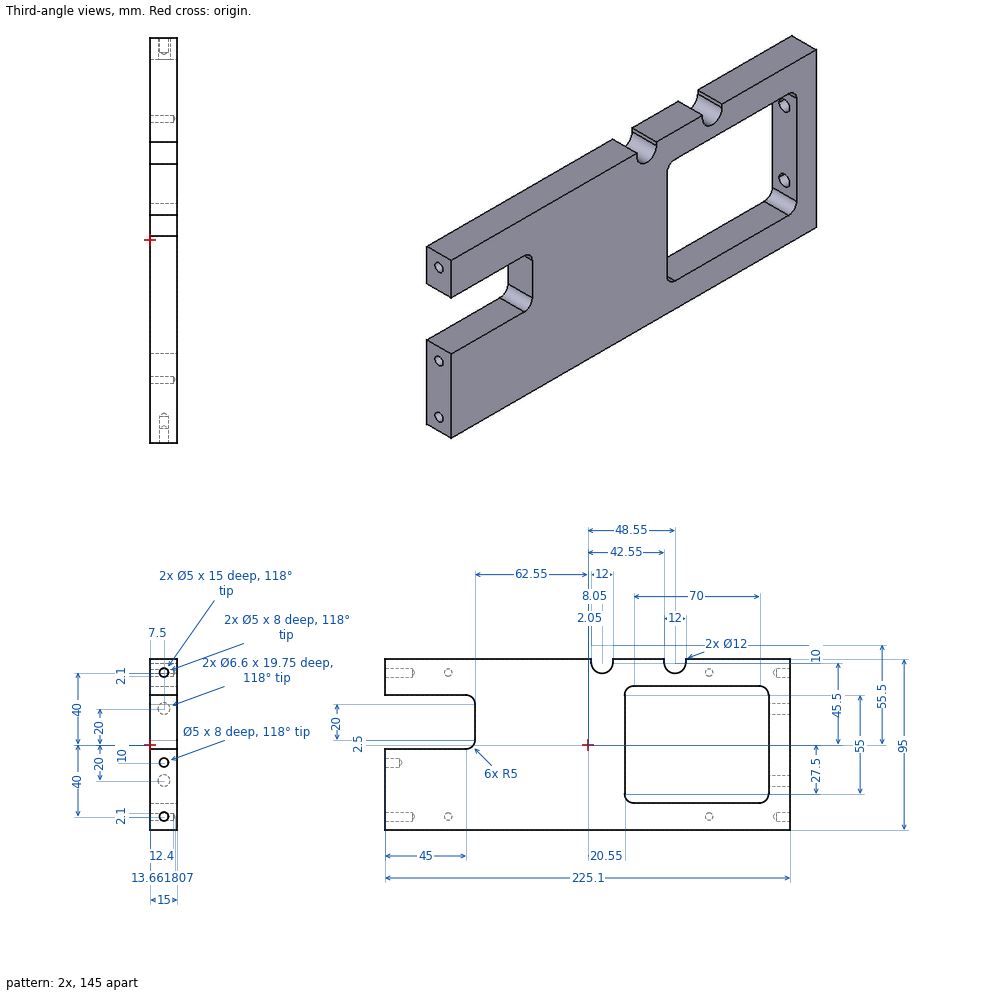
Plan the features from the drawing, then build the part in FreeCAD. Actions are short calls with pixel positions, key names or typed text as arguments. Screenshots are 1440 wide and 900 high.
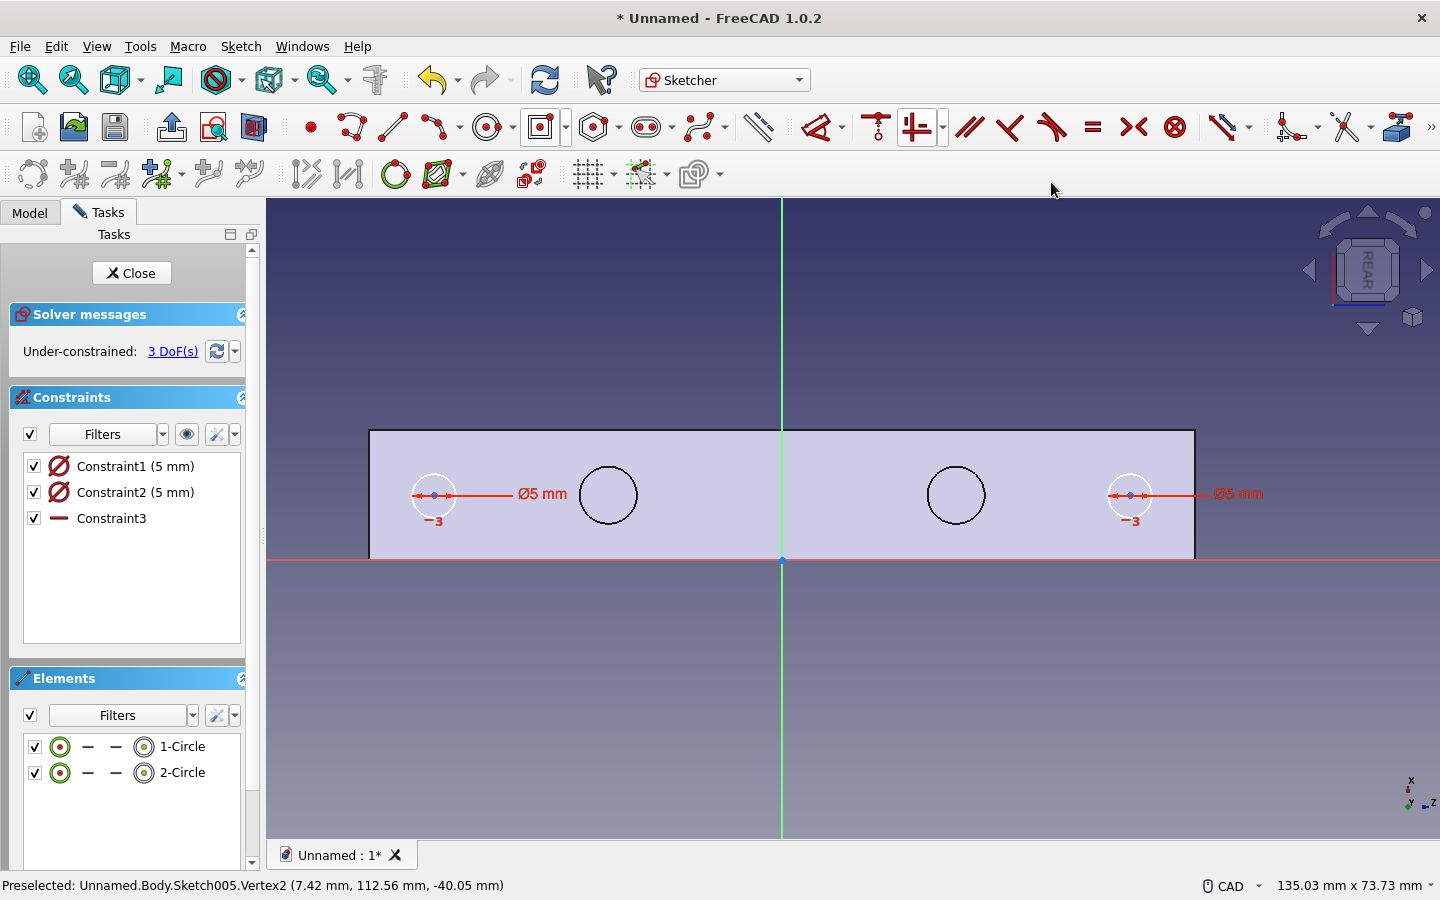
click(816, 128)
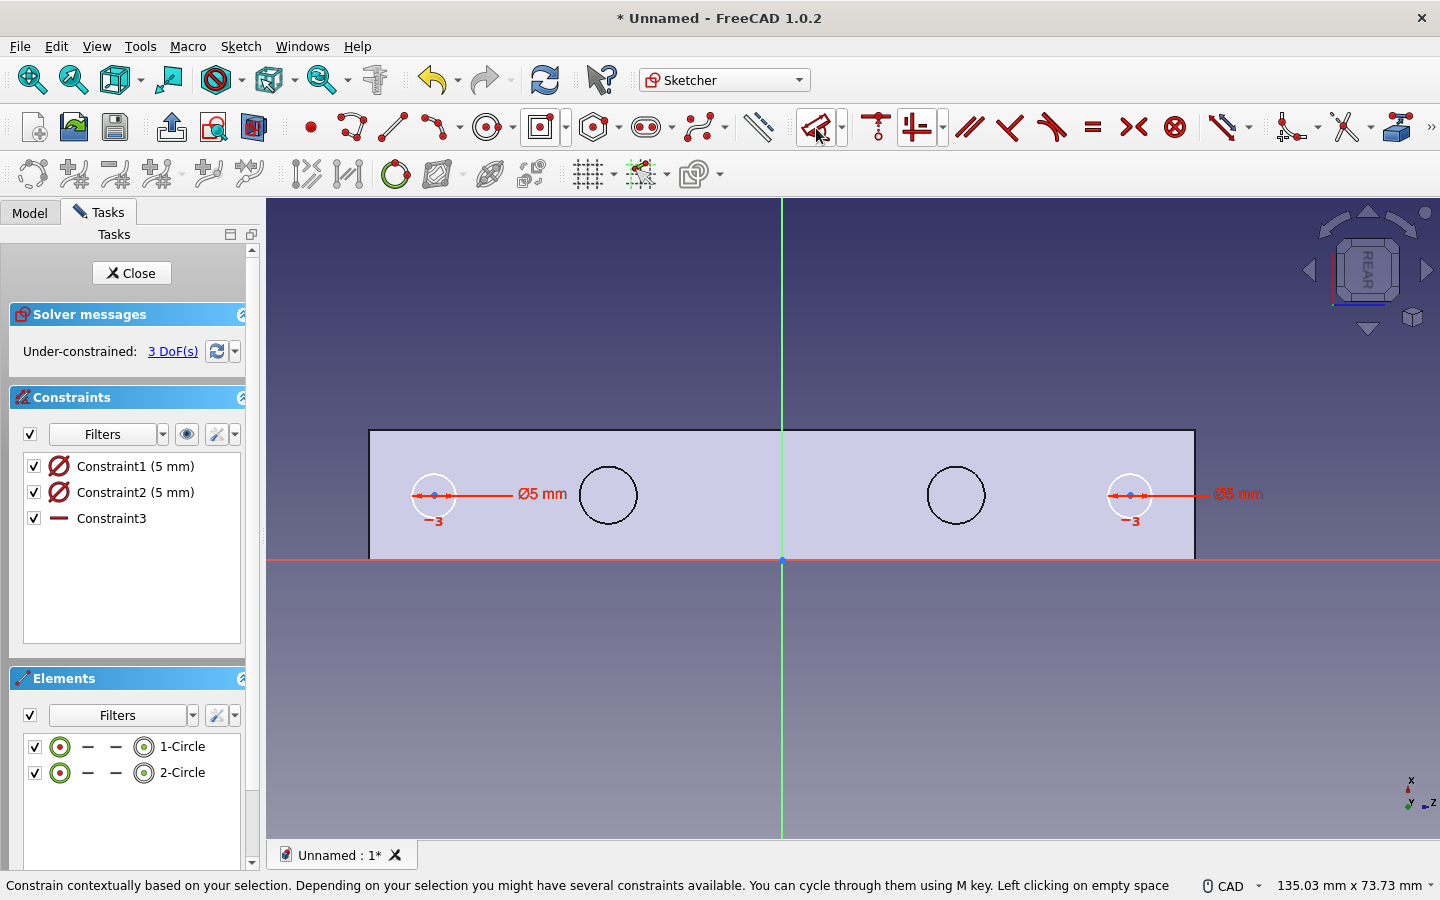
click(1130, 496)
click(956, 594)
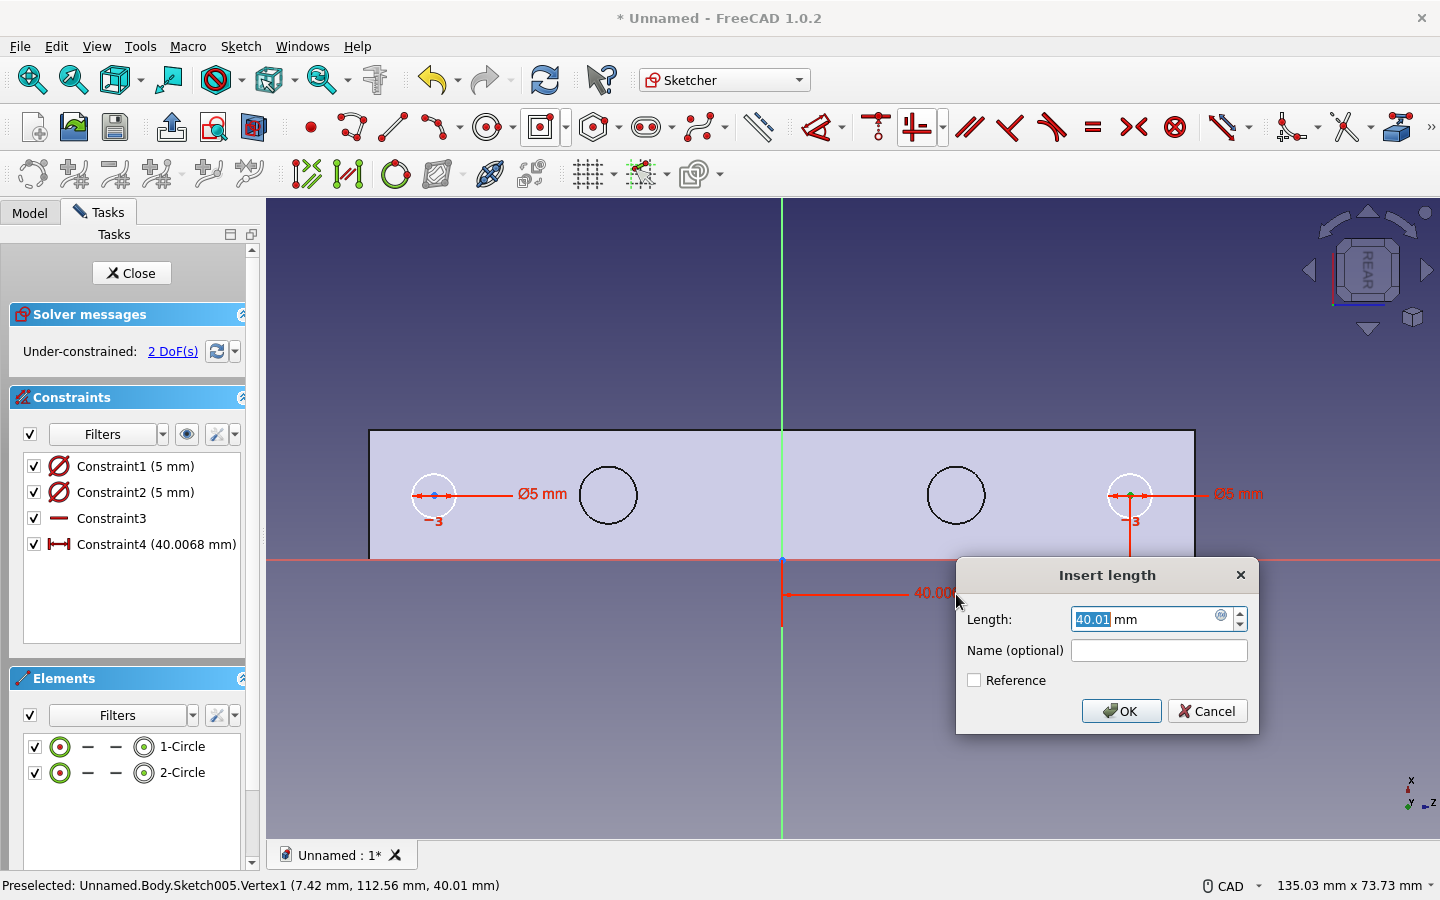
text(40)
key(Return)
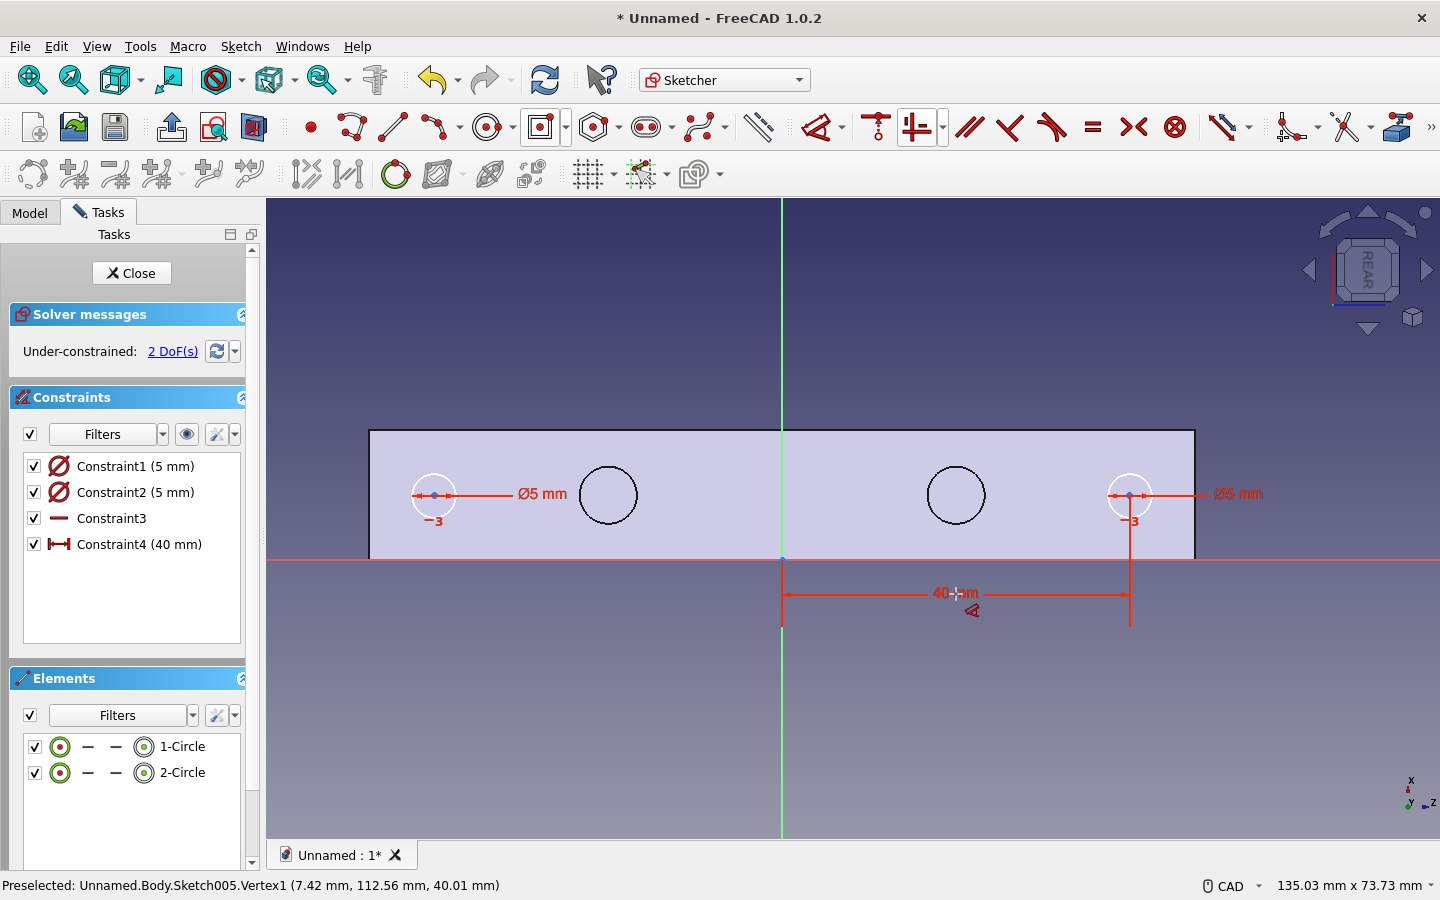
click(434, 496)
click(608, 594)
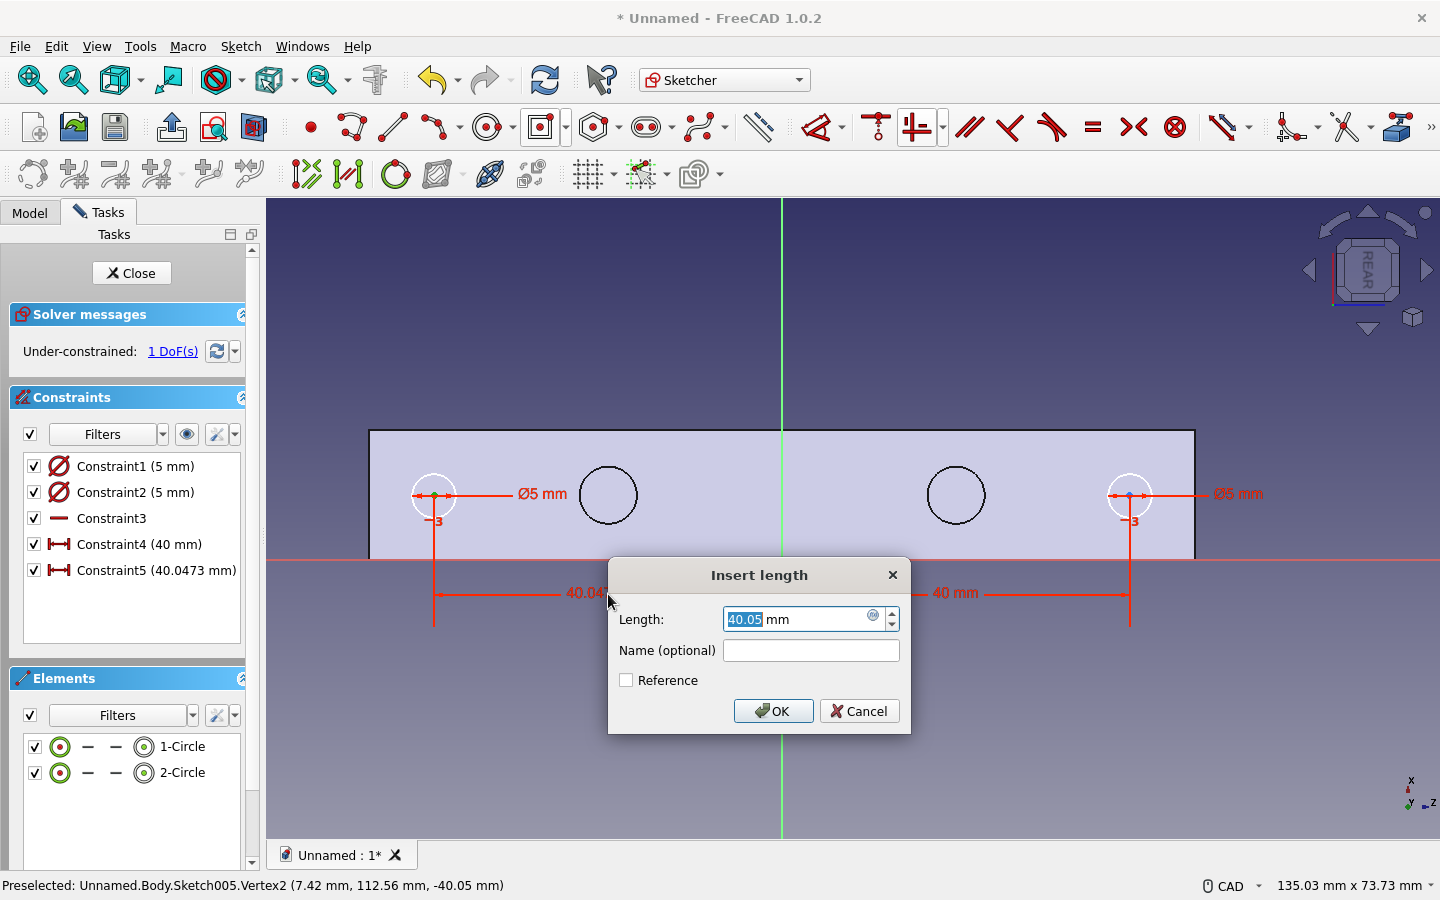
text(40)
key(Return)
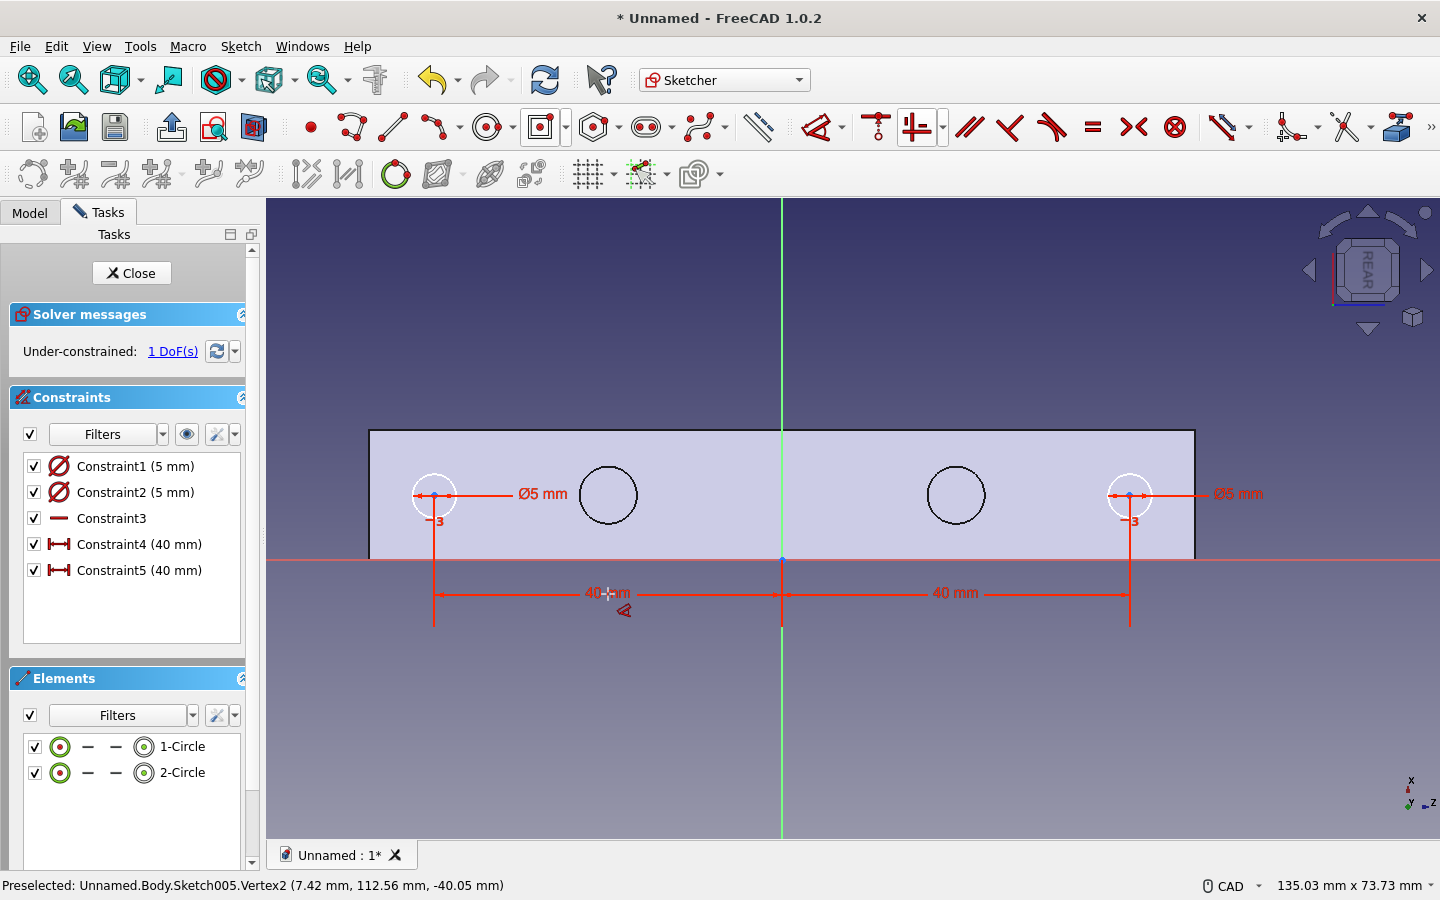
click(1130, 496)
click(1164, 528)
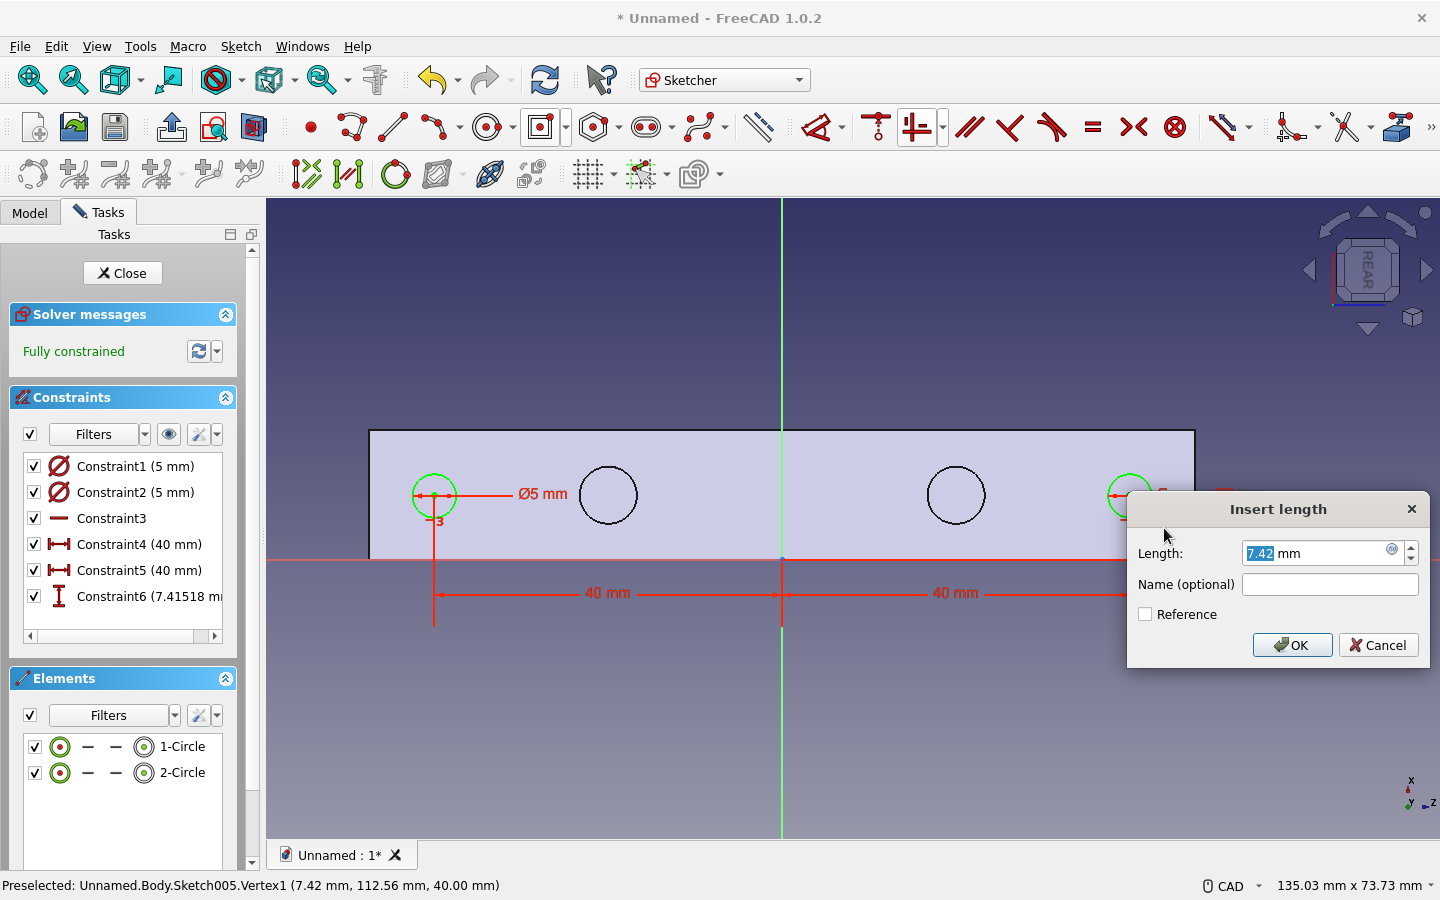
text(7.5)
key(Return)
key(Escape)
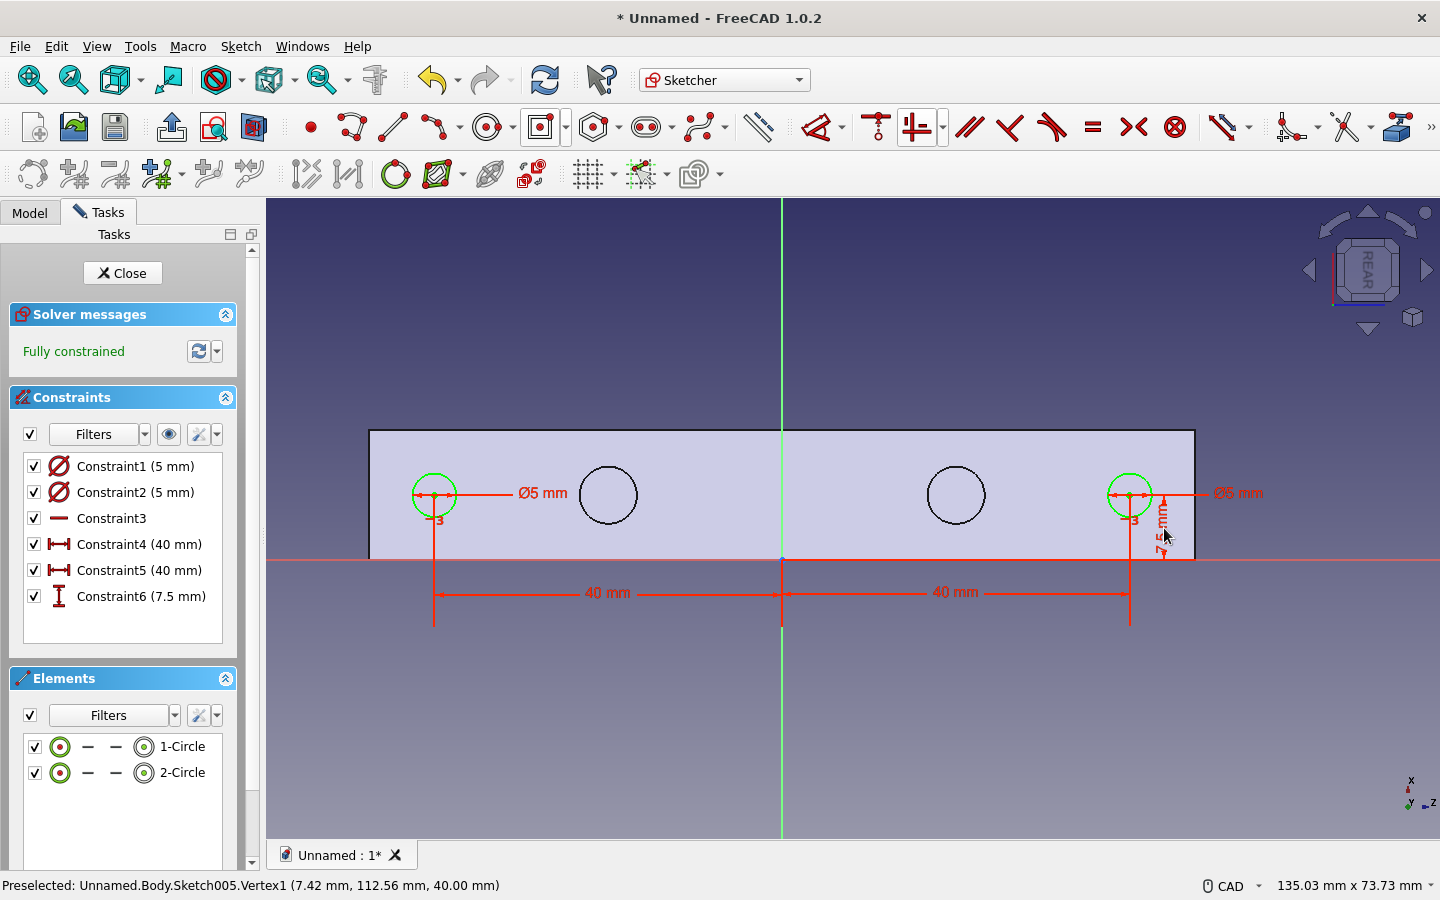
click(123, 273)